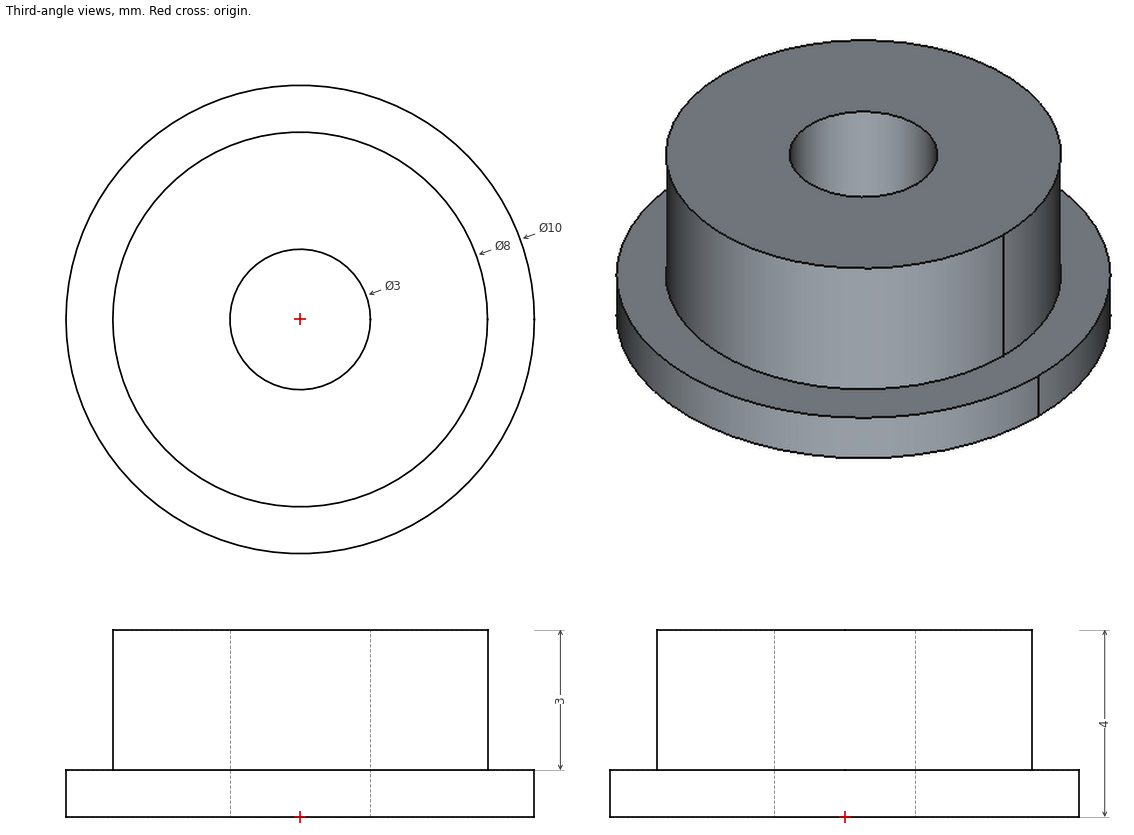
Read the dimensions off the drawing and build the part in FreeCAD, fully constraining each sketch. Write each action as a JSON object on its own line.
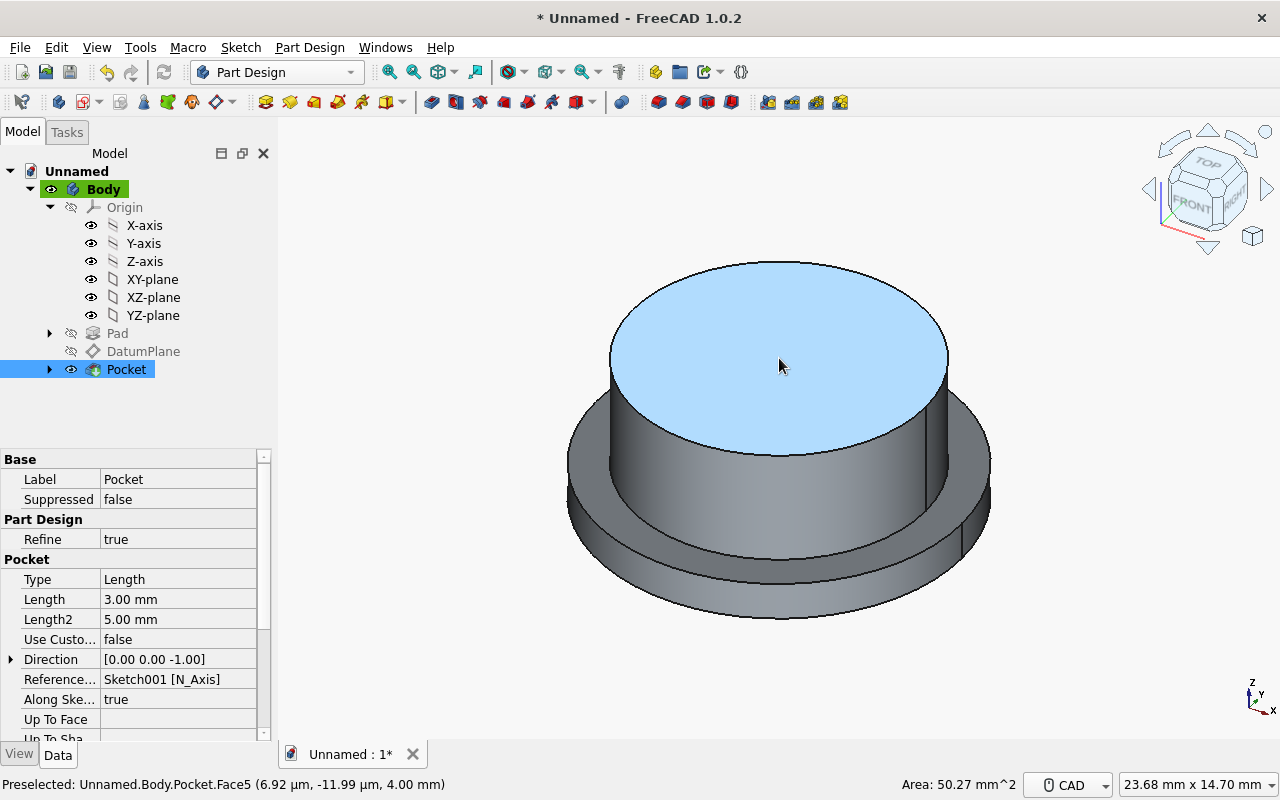
{"action": "left_click", "coordinate": [84, 102]}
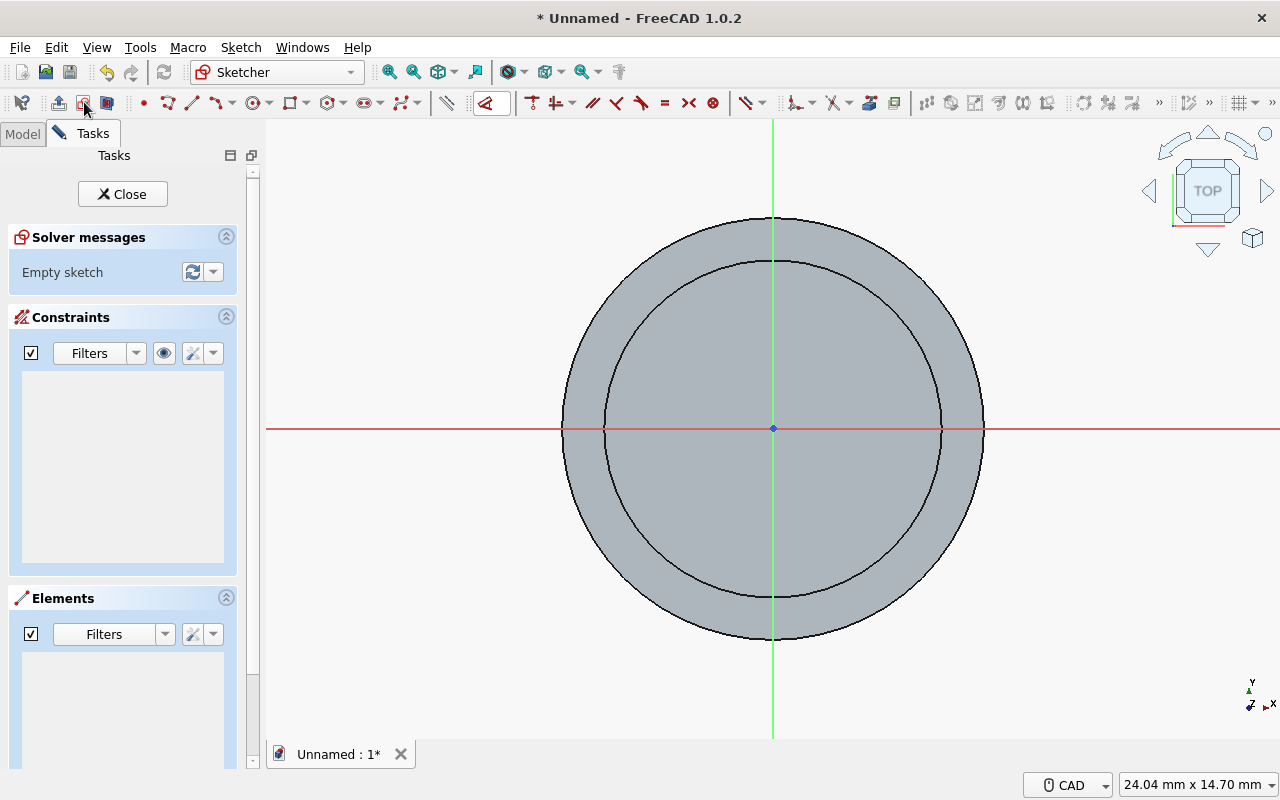
{"action": "scroll", "coordinate": [803, 429], "scroll_direction": "up", "scroll_amount": 6}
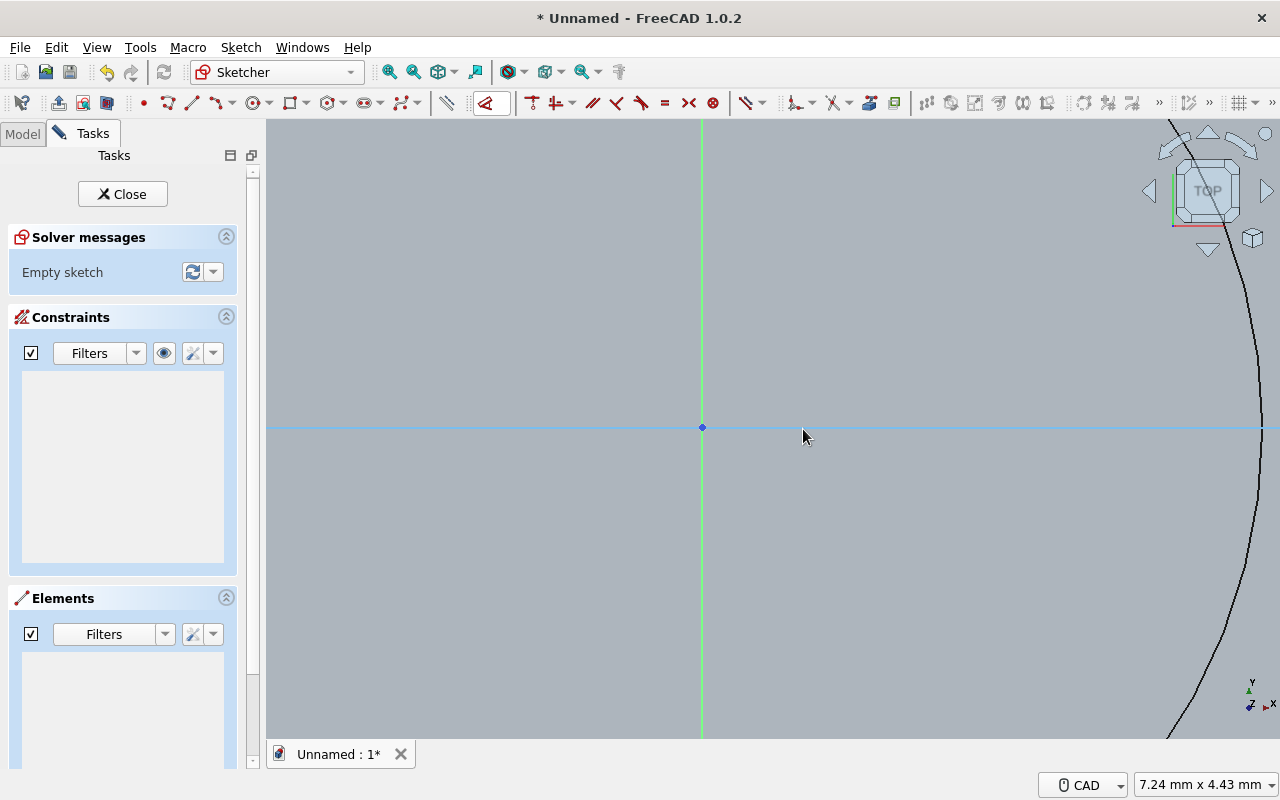
{"action": "key", "text": "g c"}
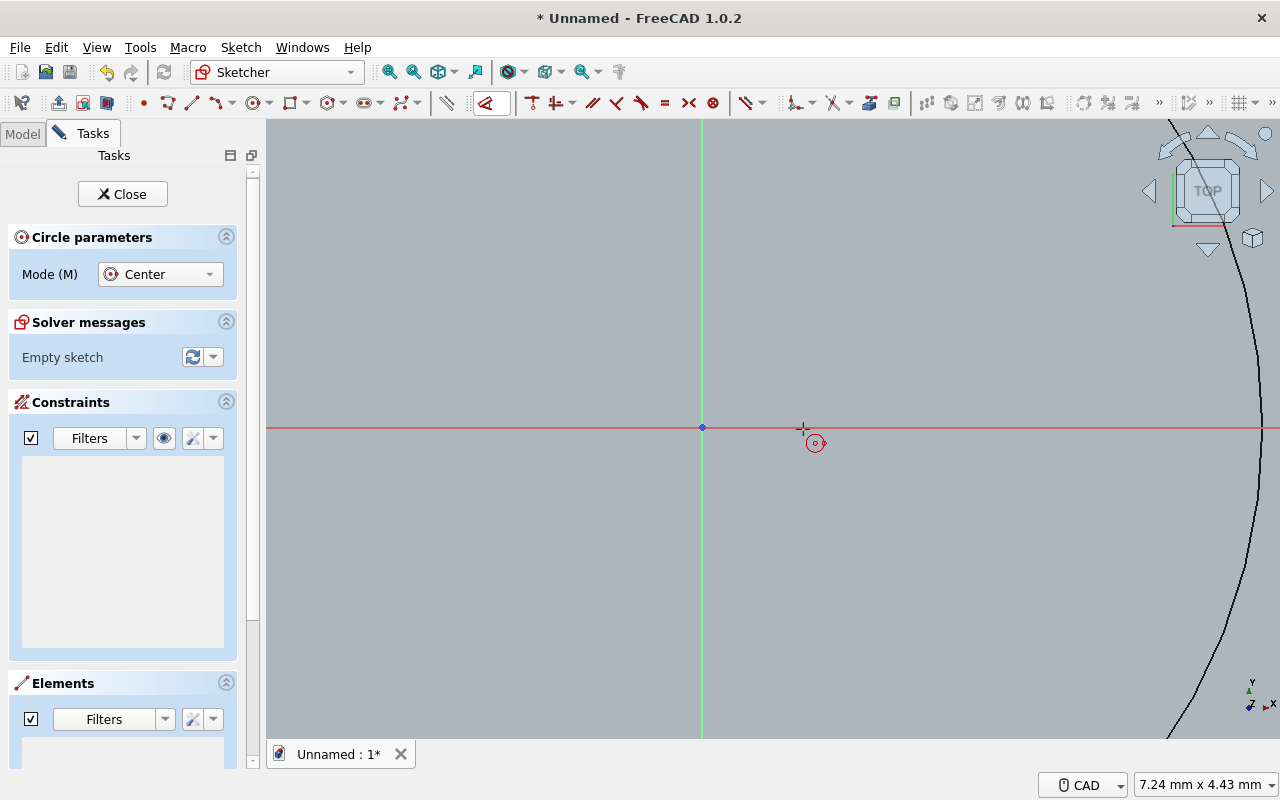
{"action": "left_click", "coordinate": [702, 428]}
{"action": "left_click", "coordinate": [851, 279]}
{"action": "key", "text": "Escape"}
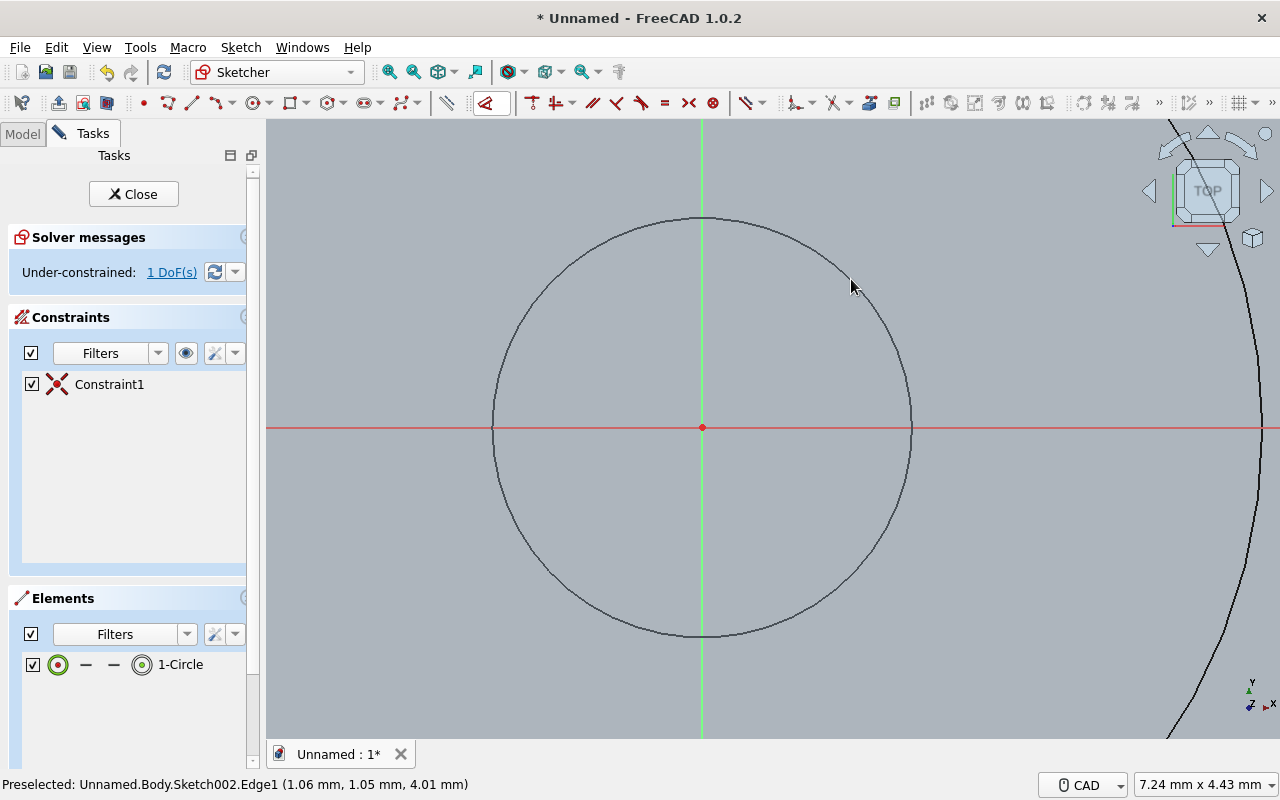
{"action": "left_click", "coordinate": [850, 279]}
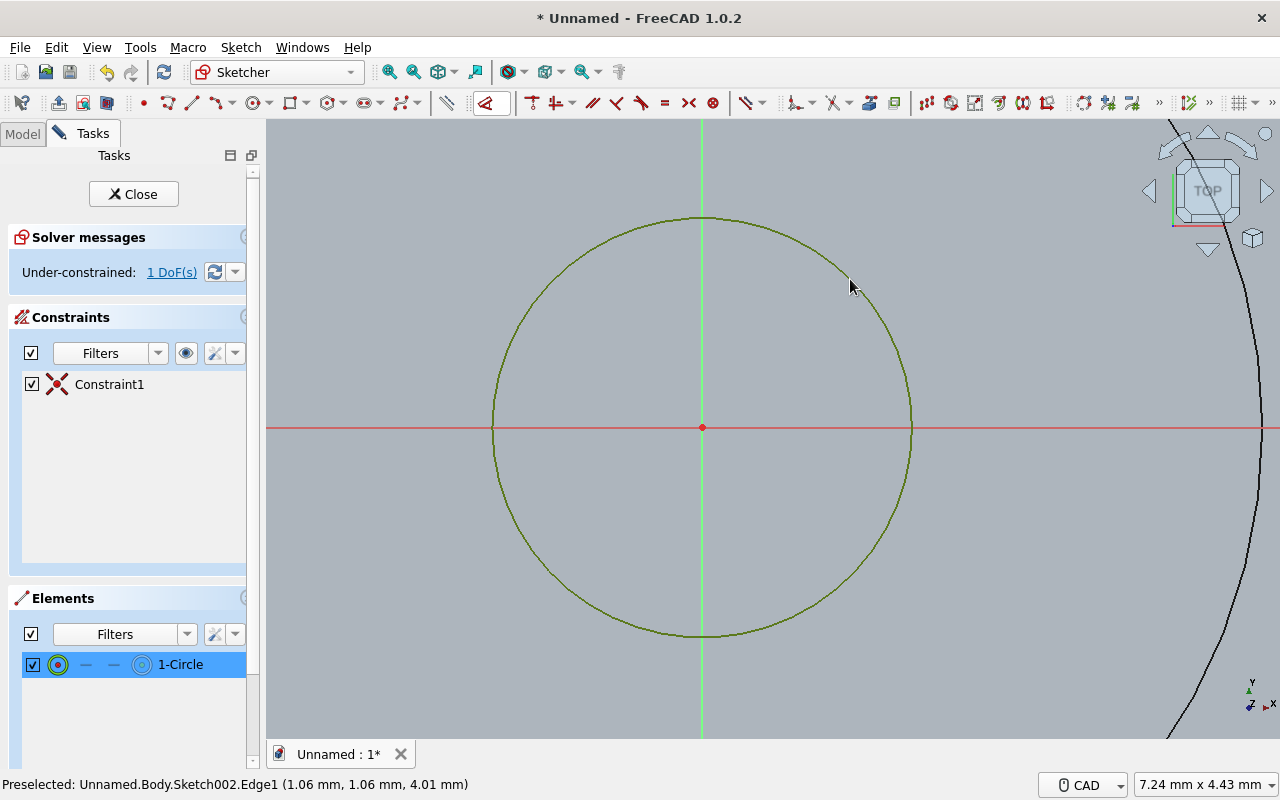
{"action": "key", "text": "k o"}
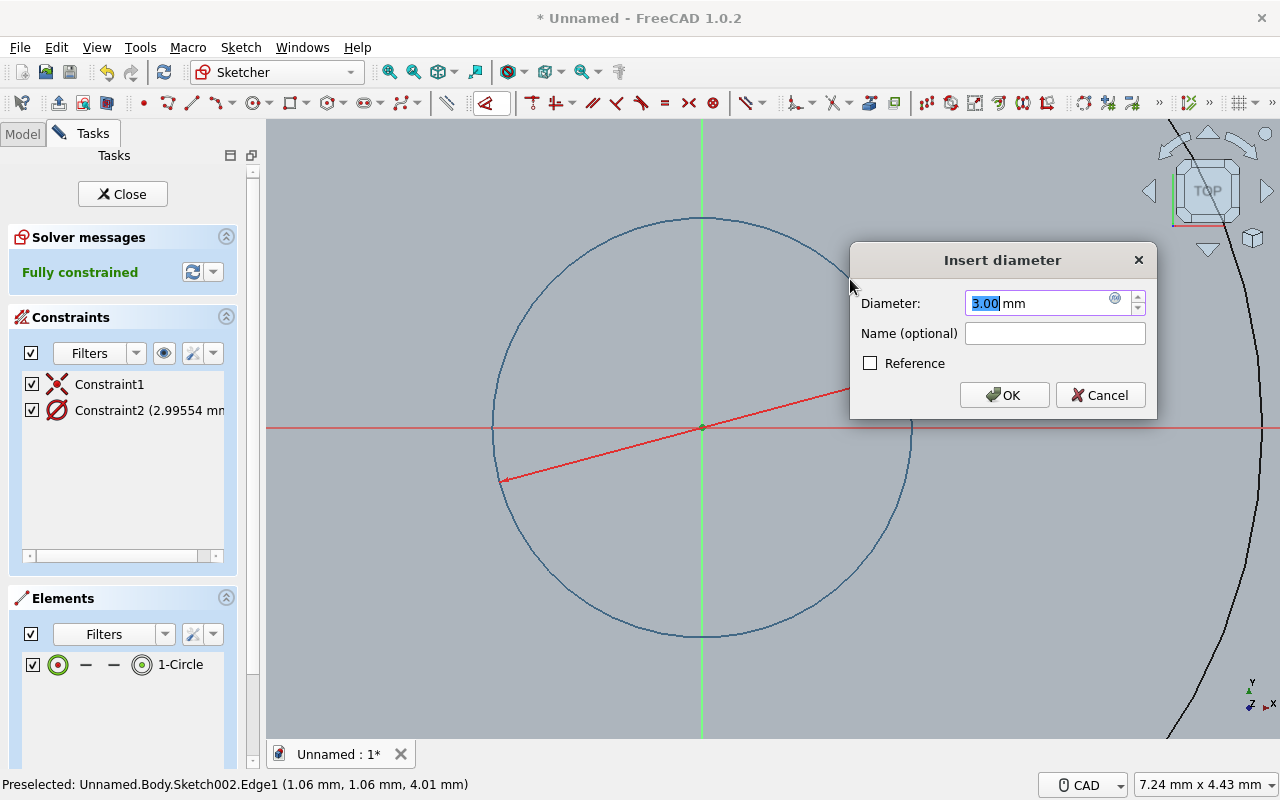
{"action": "type", "text": "3"}
{"action": "key", "text": "Return"}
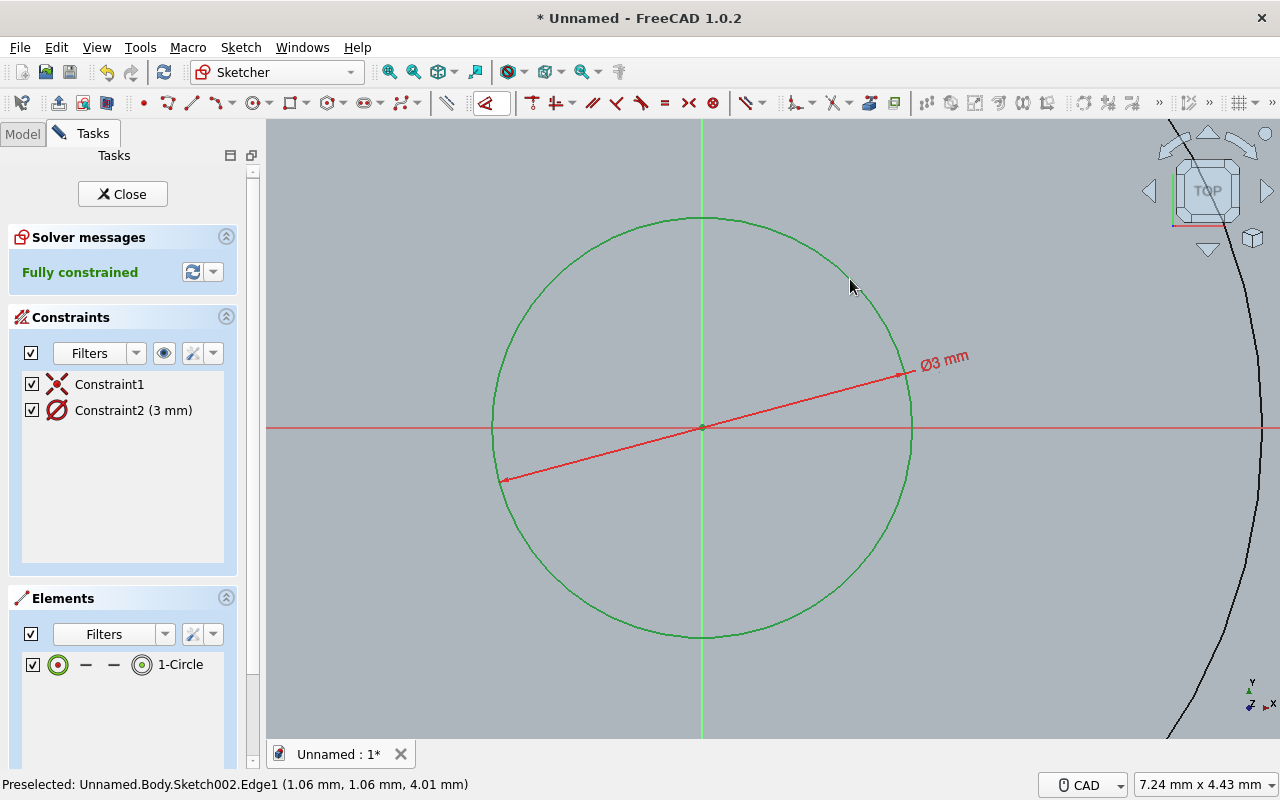
{"action": "left_click", "coordinate": [123, 194]}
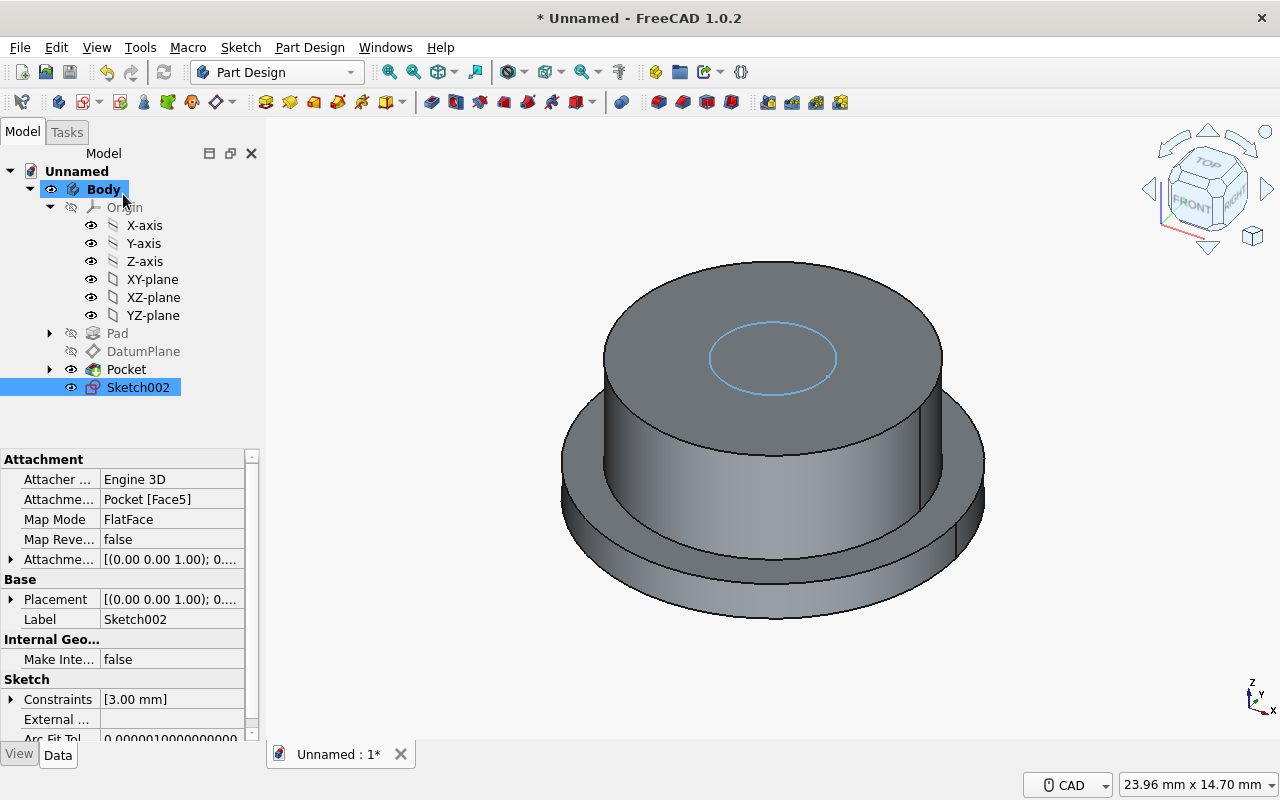
{"action": "left_click", "coordinate": [432, 102]}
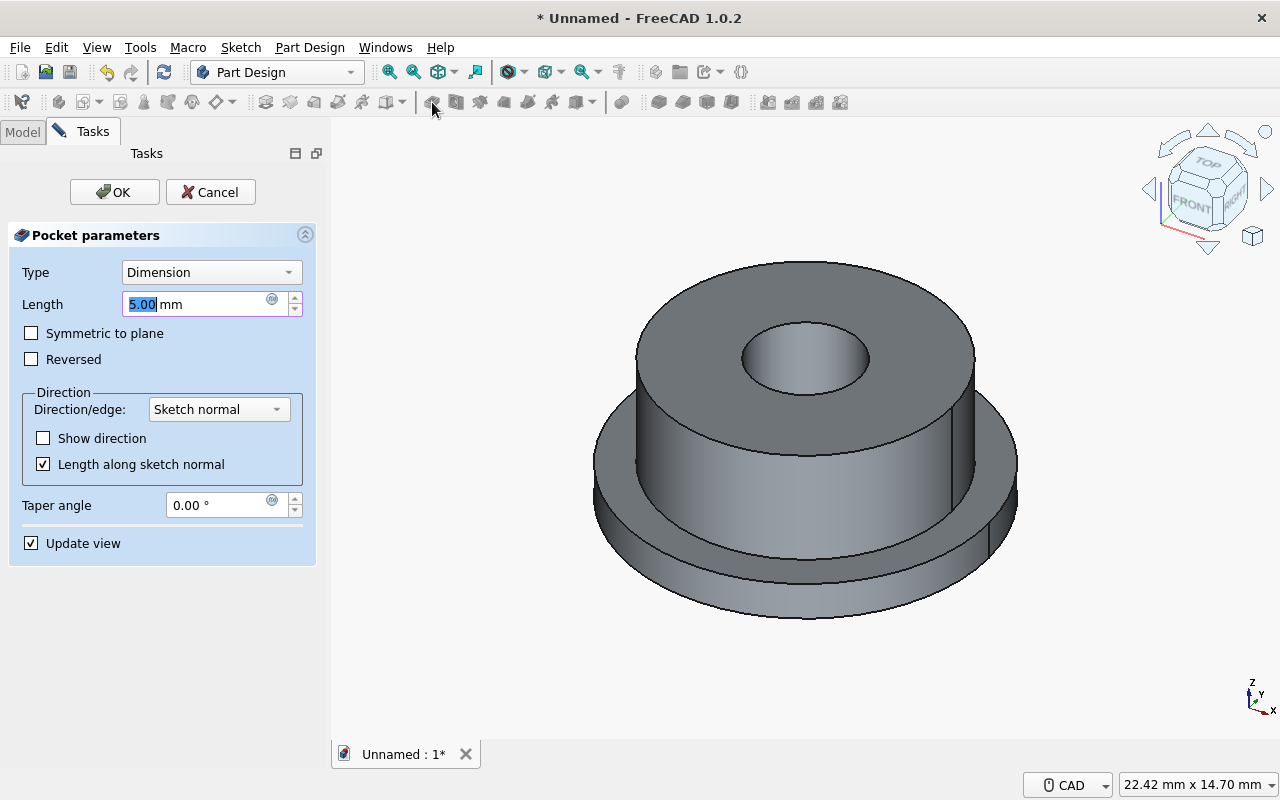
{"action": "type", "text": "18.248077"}
{"action": "key", "text": "Tab"}